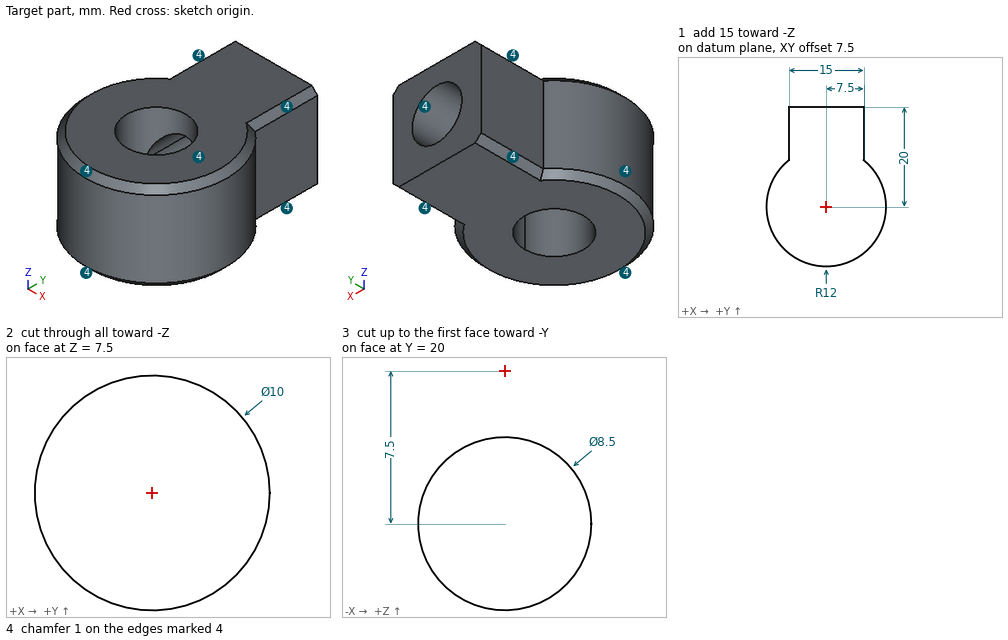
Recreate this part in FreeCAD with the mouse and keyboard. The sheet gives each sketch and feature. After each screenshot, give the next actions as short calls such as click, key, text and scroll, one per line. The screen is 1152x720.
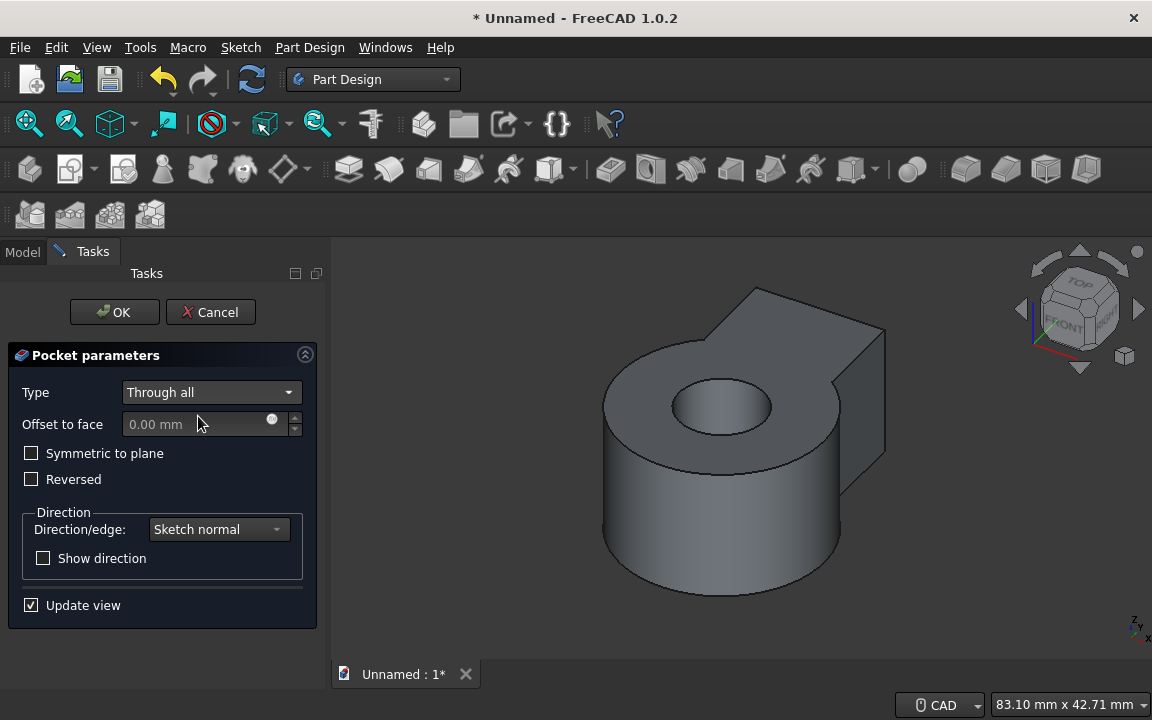
click(115, 312)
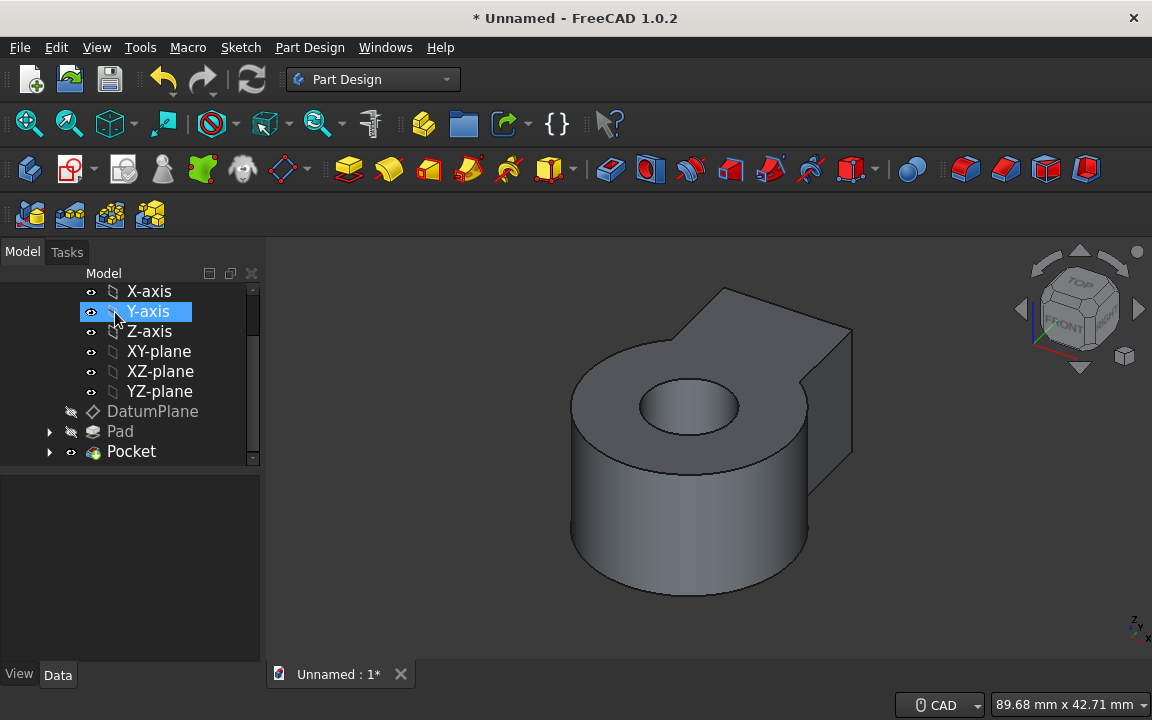
key(4)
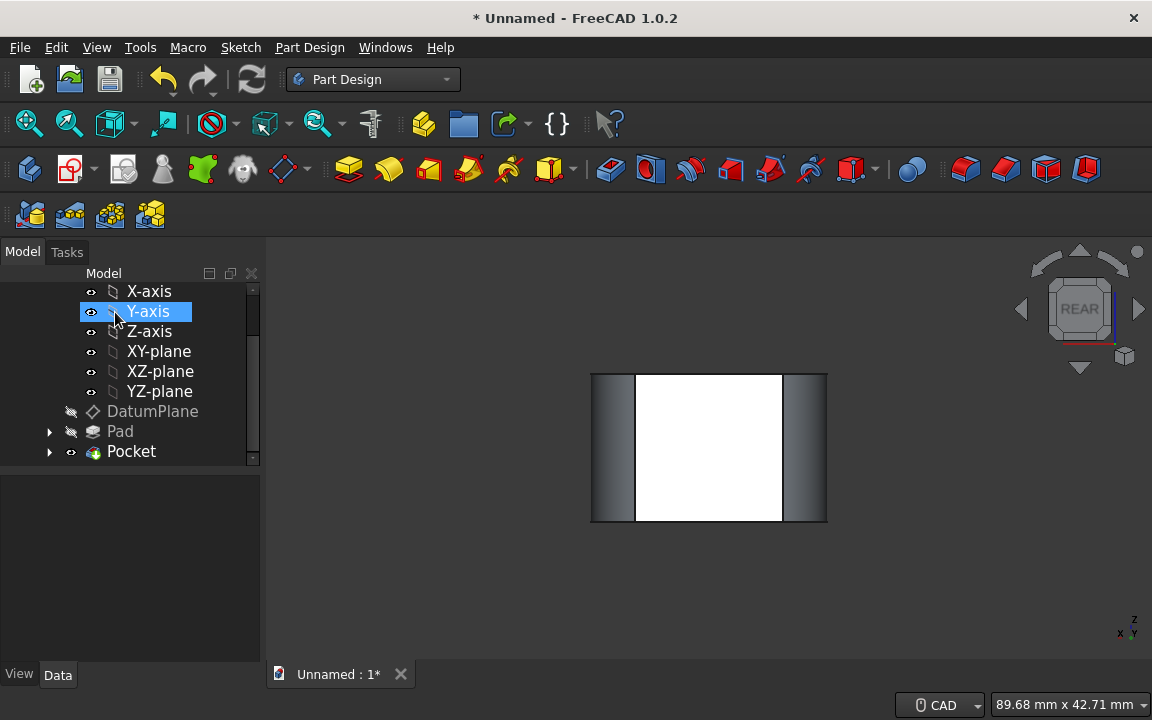
click(30, 124)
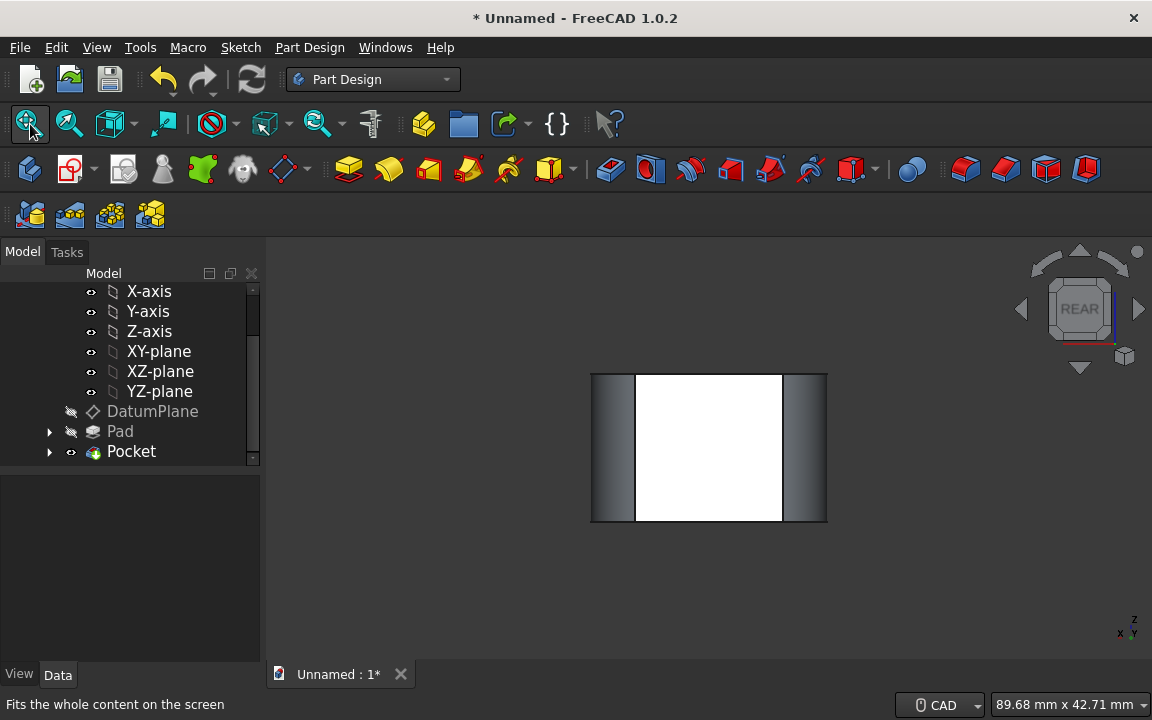
click(709, 447)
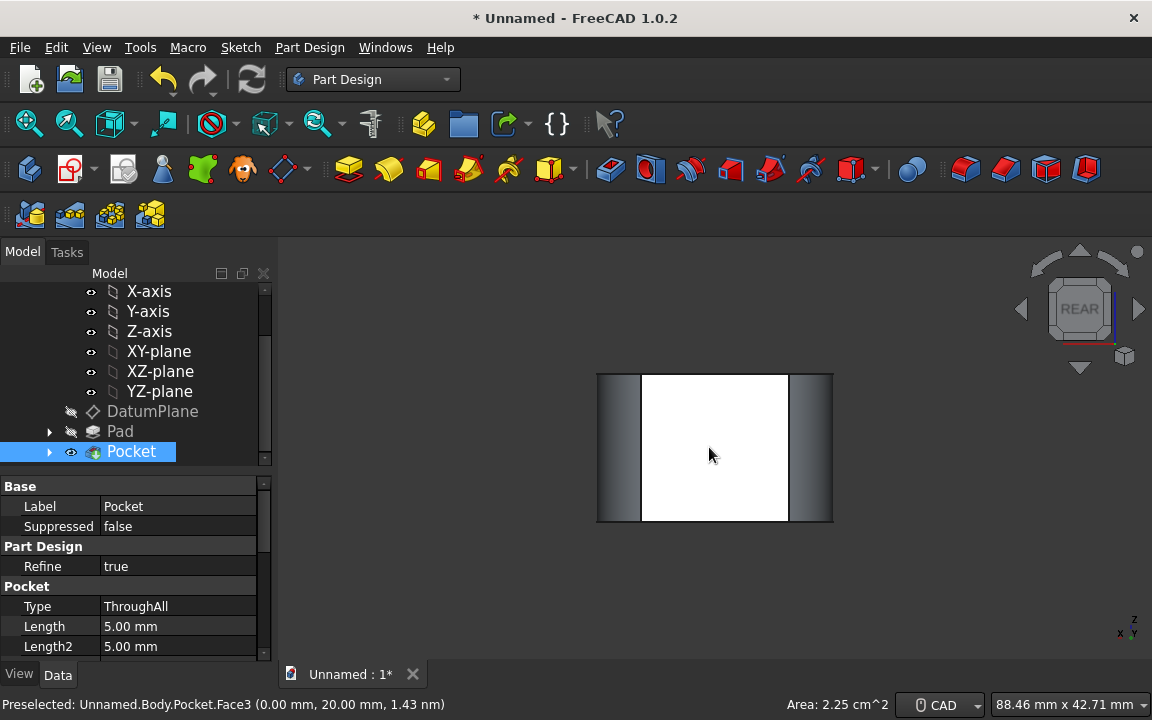
click(70, 170)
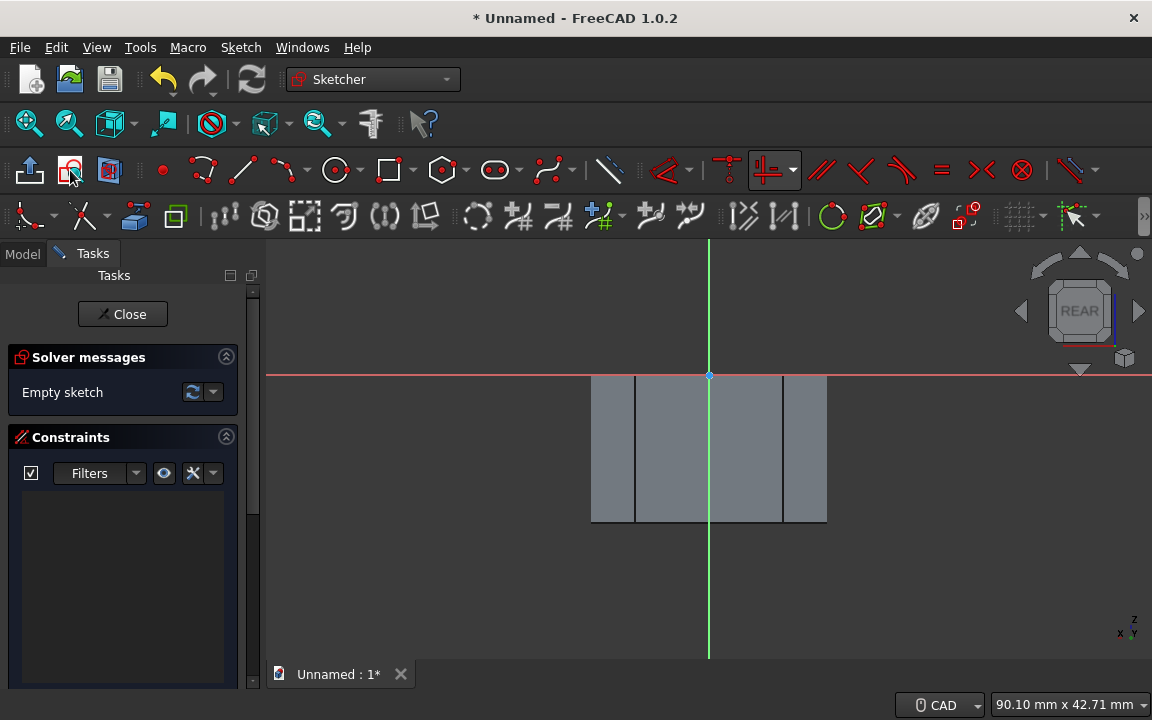
scroll(765, 420, up, 4)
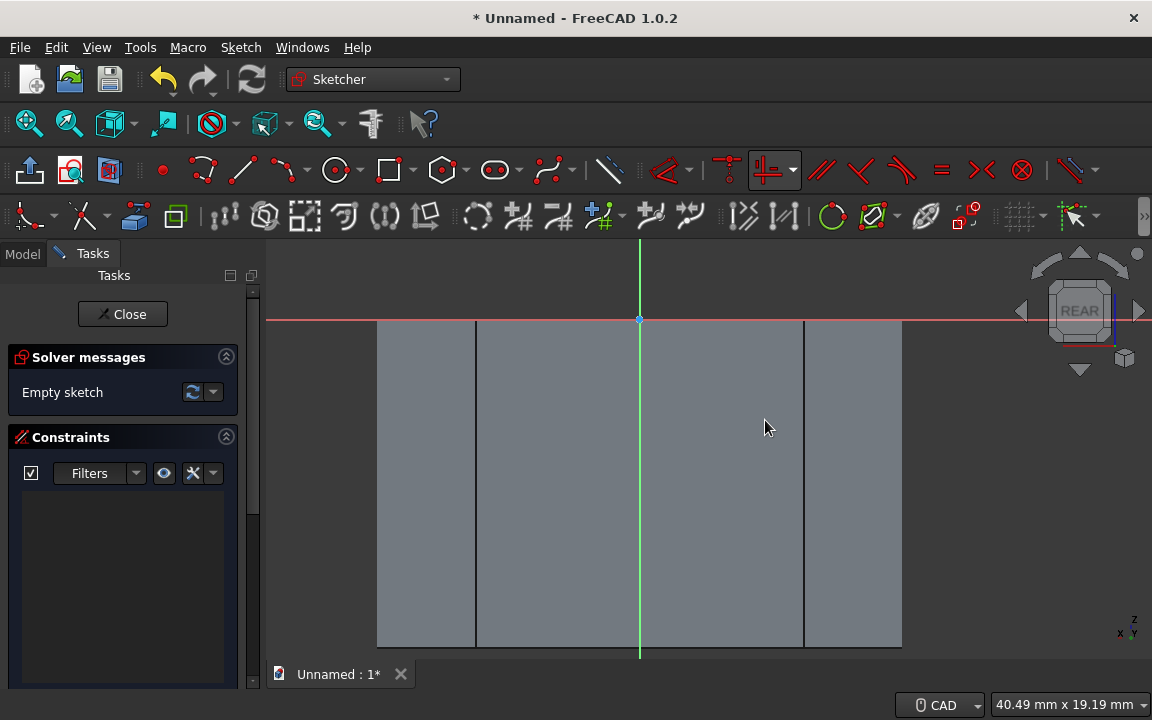
click(336, 170)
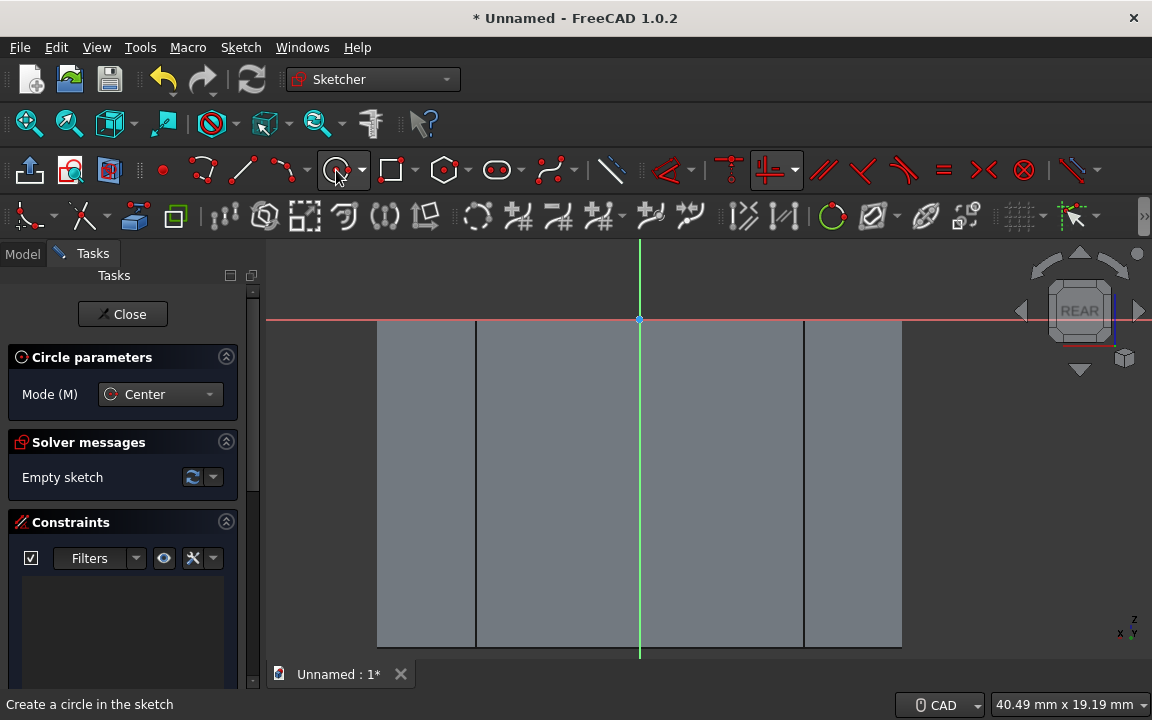
click(640, 484)
click(705, 418)
key(Escape)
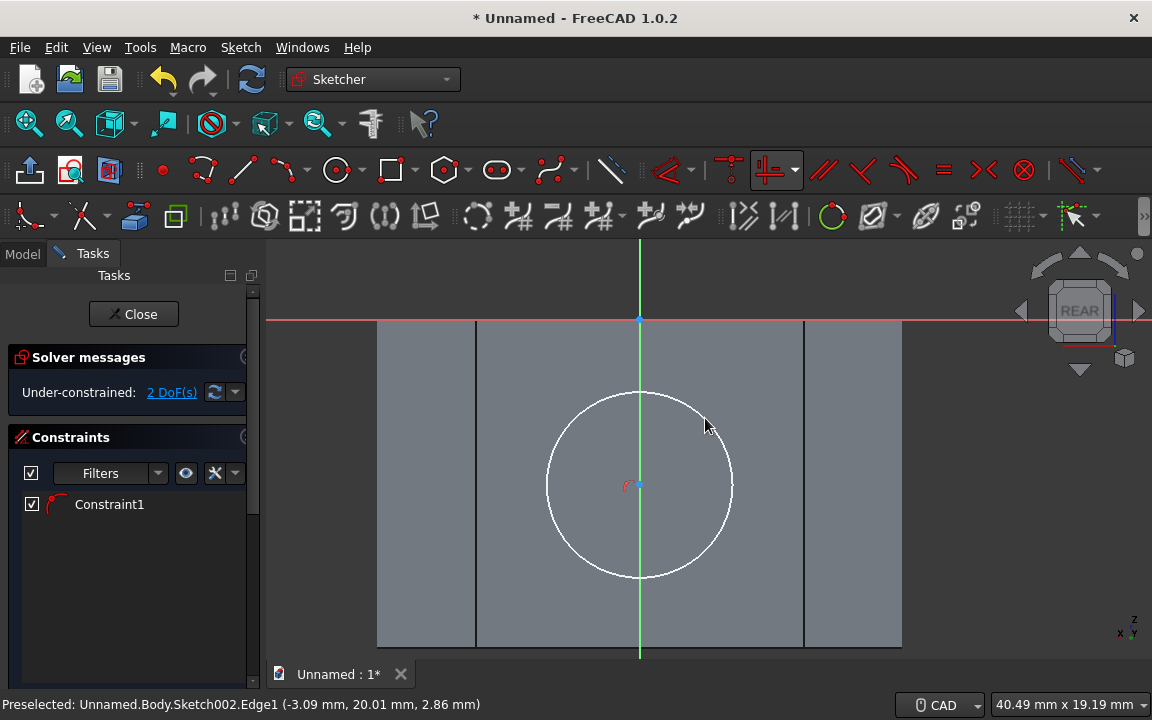
click(666, 170)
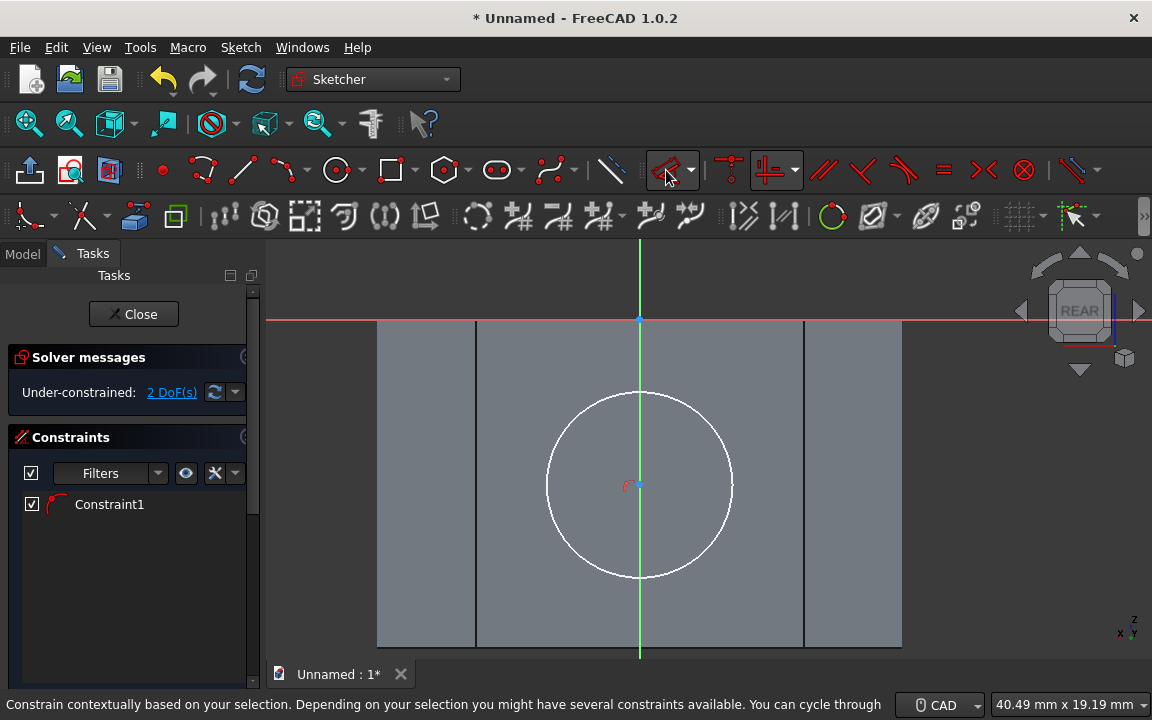
click(705, 419)
click(728, 396)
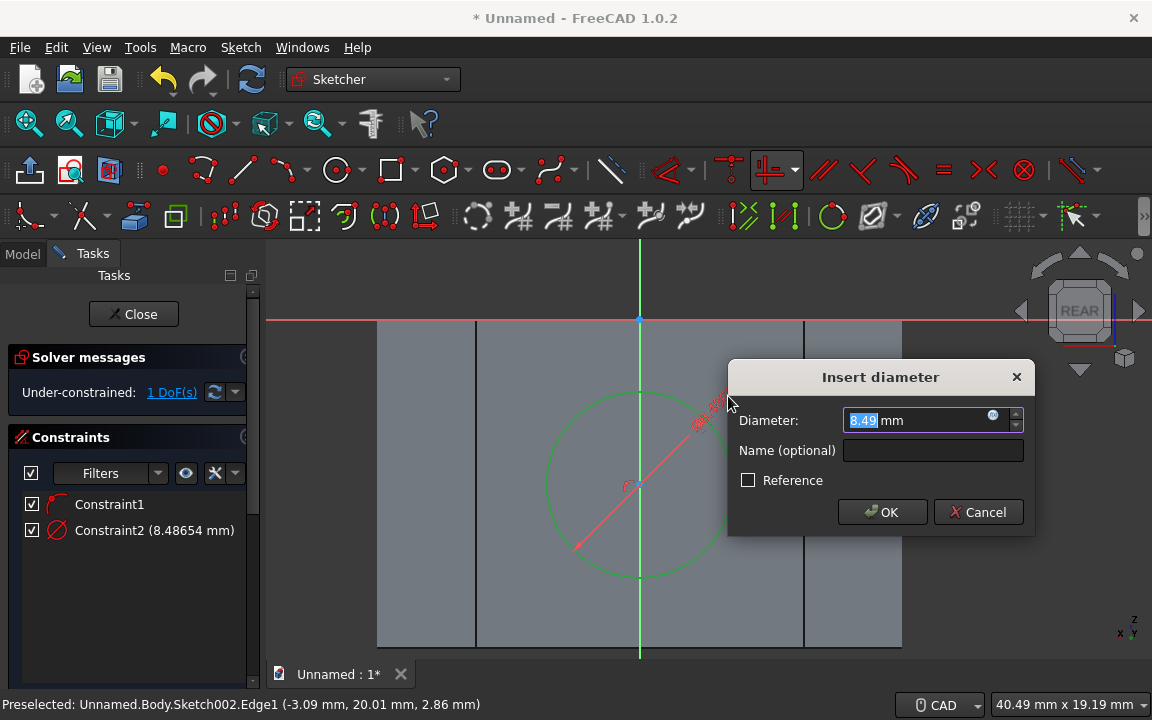
text(8.5)
key(Return)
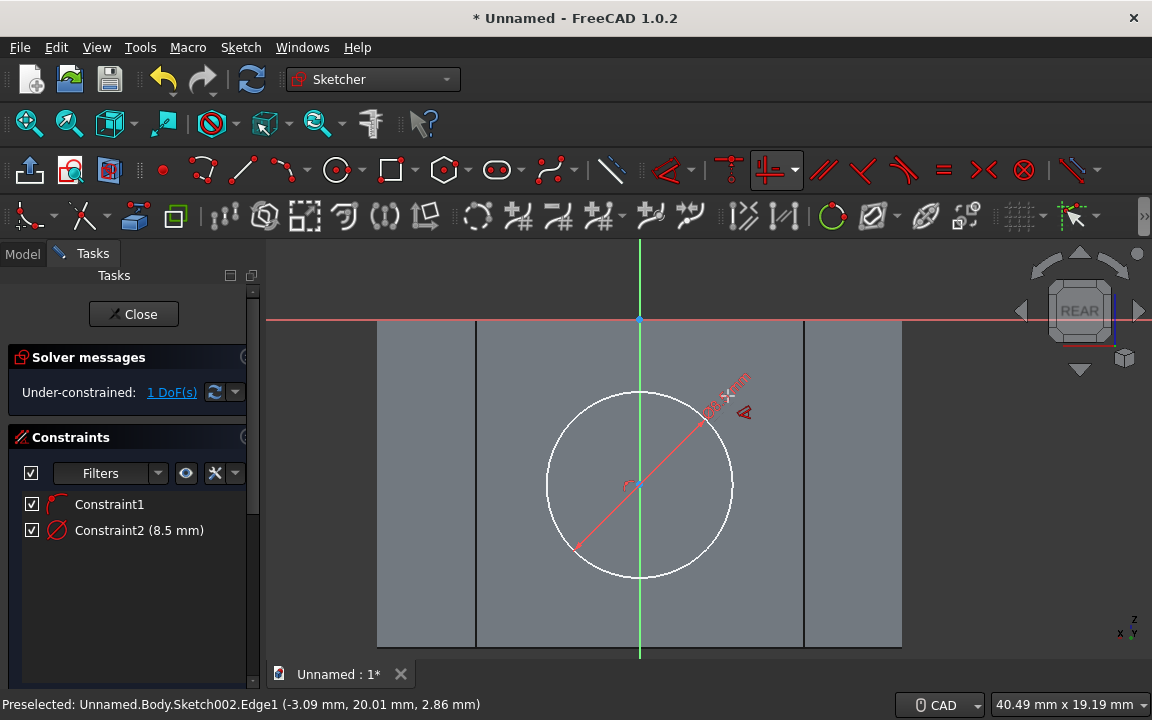
click(640, 485)
click(674, 364)